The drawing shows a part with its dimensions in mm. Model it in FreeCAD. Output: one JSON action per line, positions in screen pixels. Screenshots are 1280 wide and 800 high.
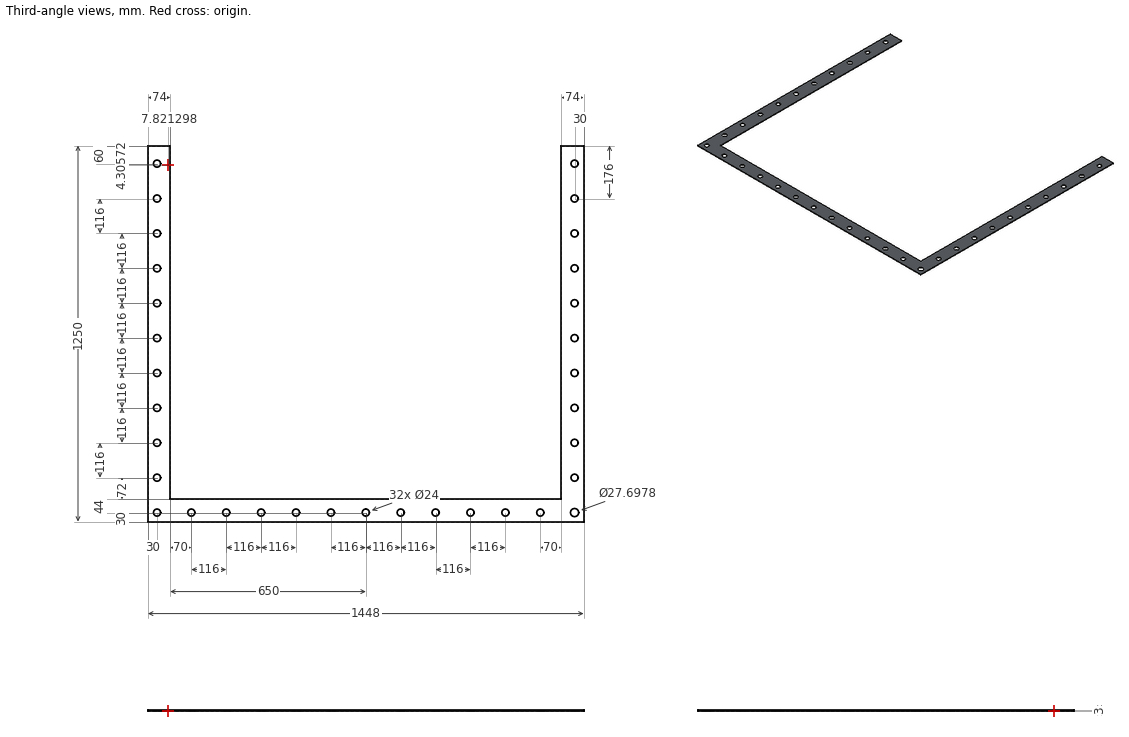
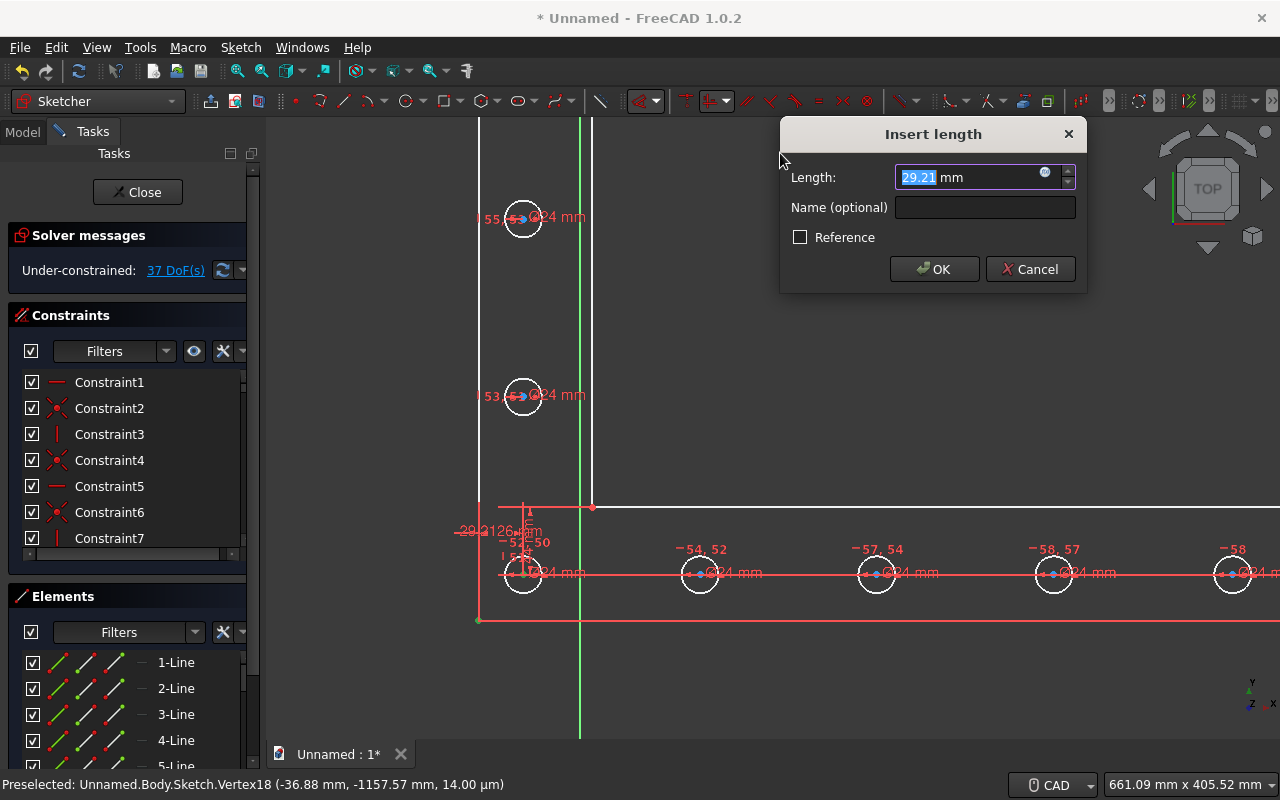
{"action": "type", "text": "30"}
{"action": "key", "text": "Return"}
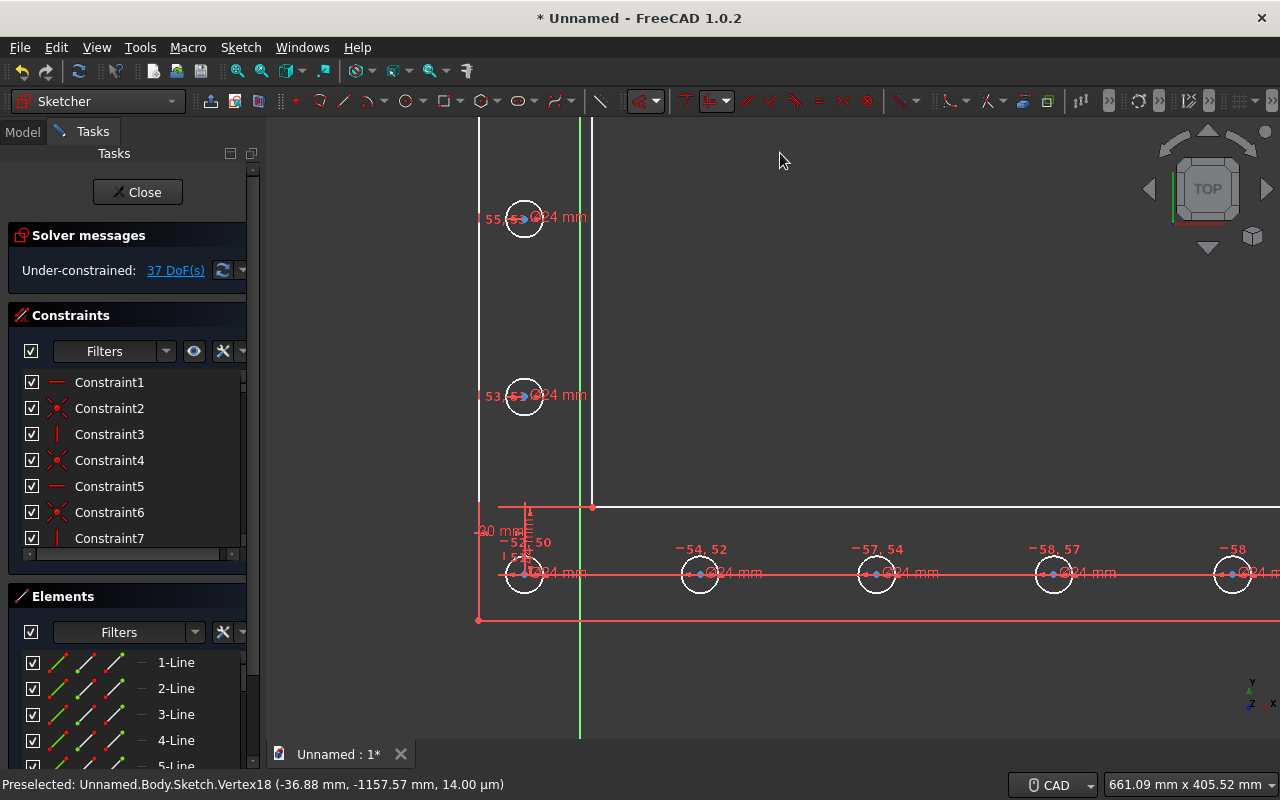
{"action": "left_click", "coordinate": [592, 507]}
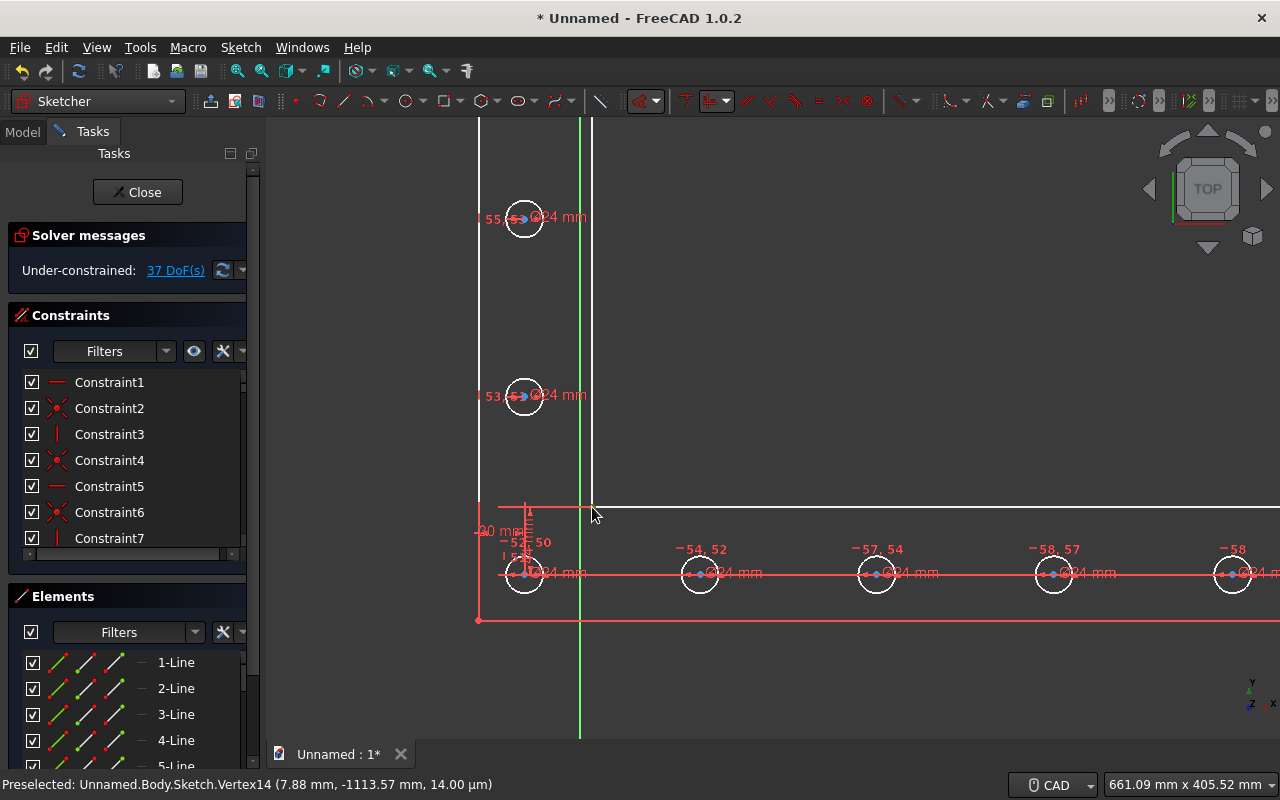
{"action": "left_click", "coordinate": [525, 397]}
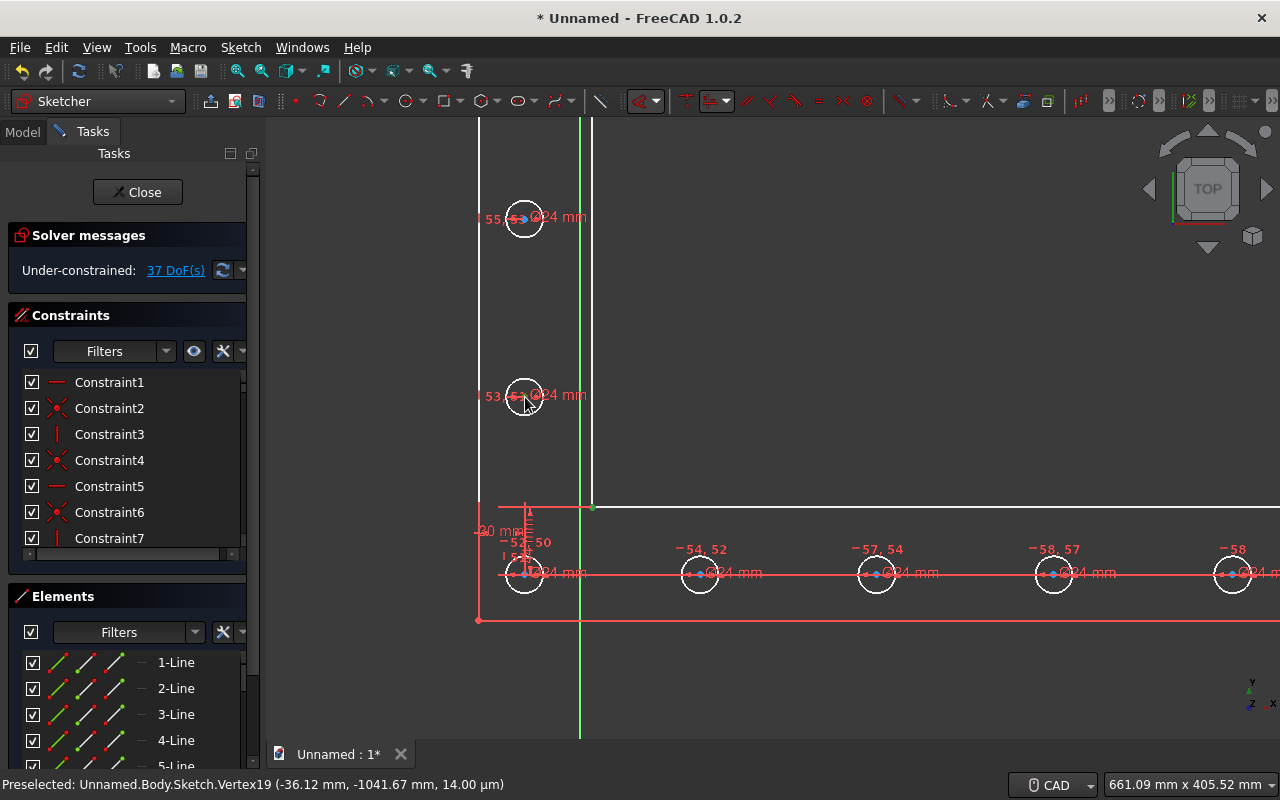
{"action": "left_click", "coordinate": [658, 102]}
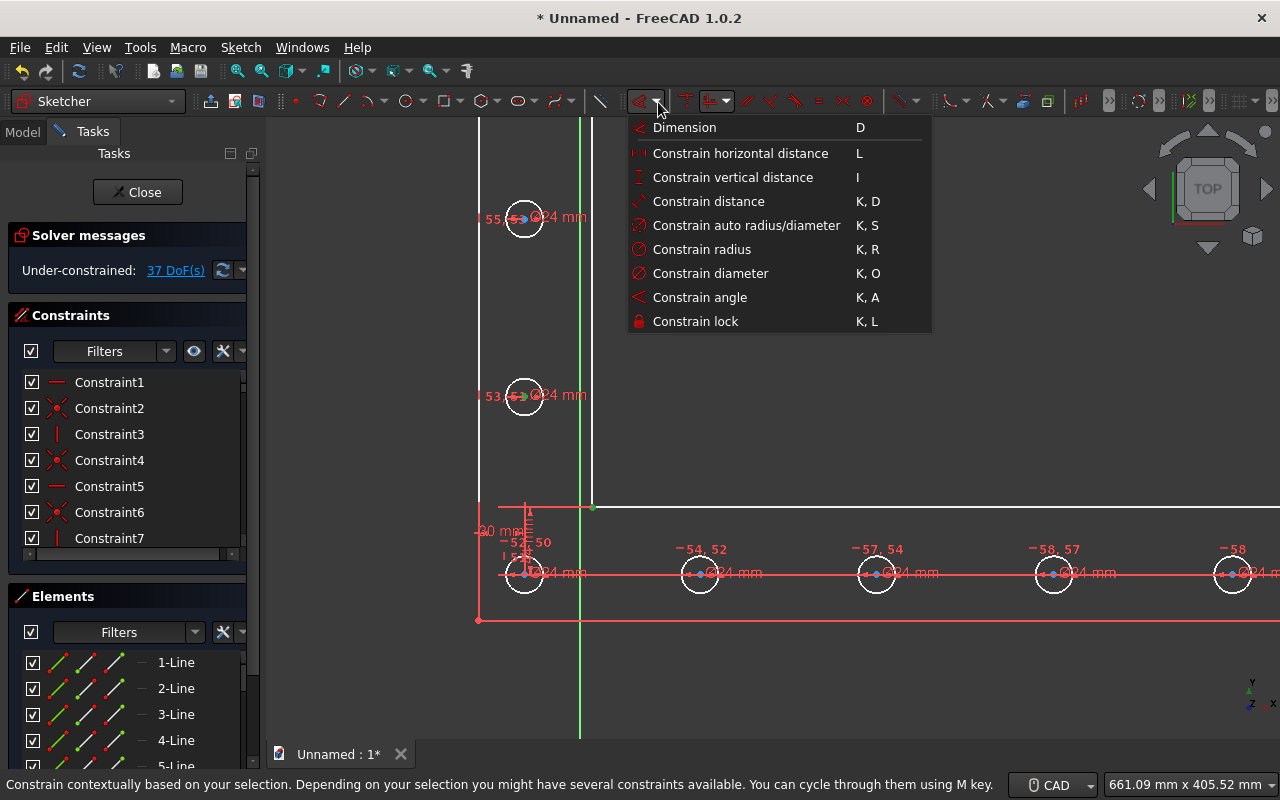
{"action": "left_click", "coordinate": [780, 177]}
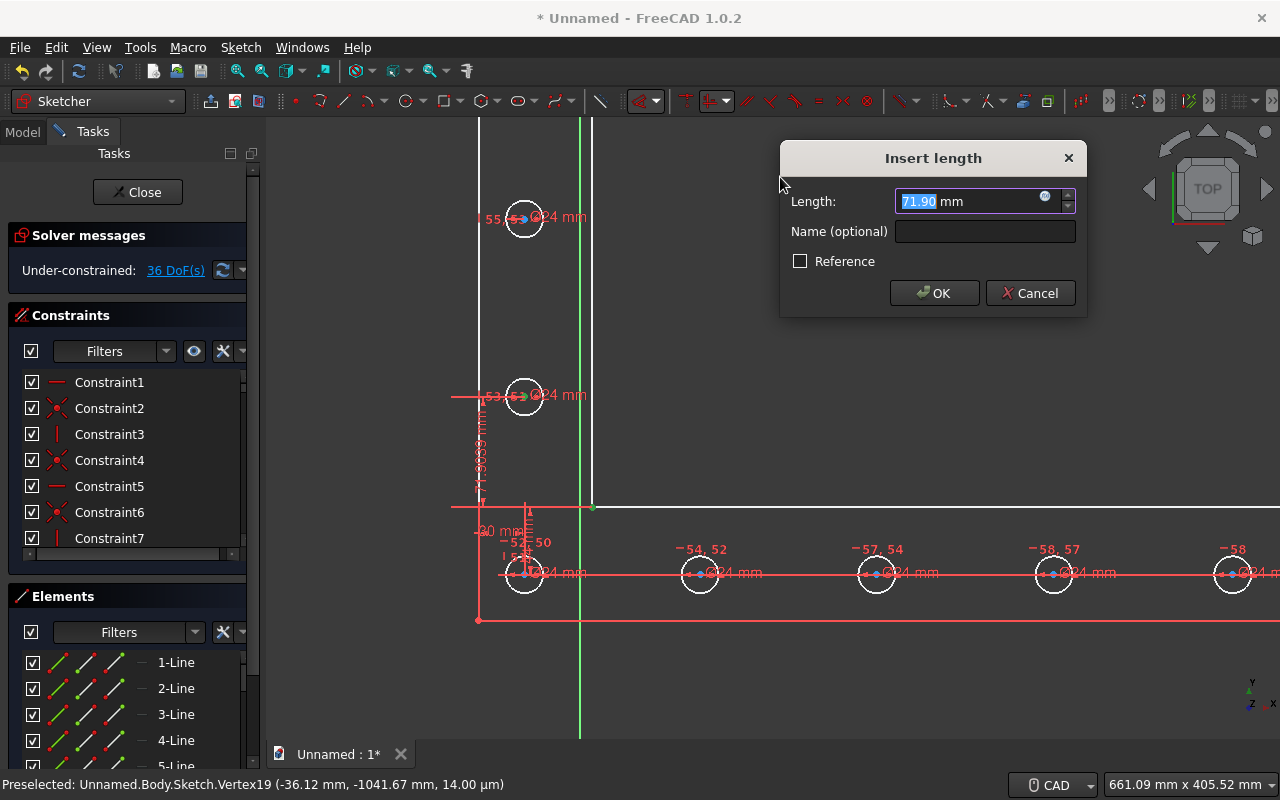
{"action": "type", "text": "72"}
{"action": "key", "text": "Return"}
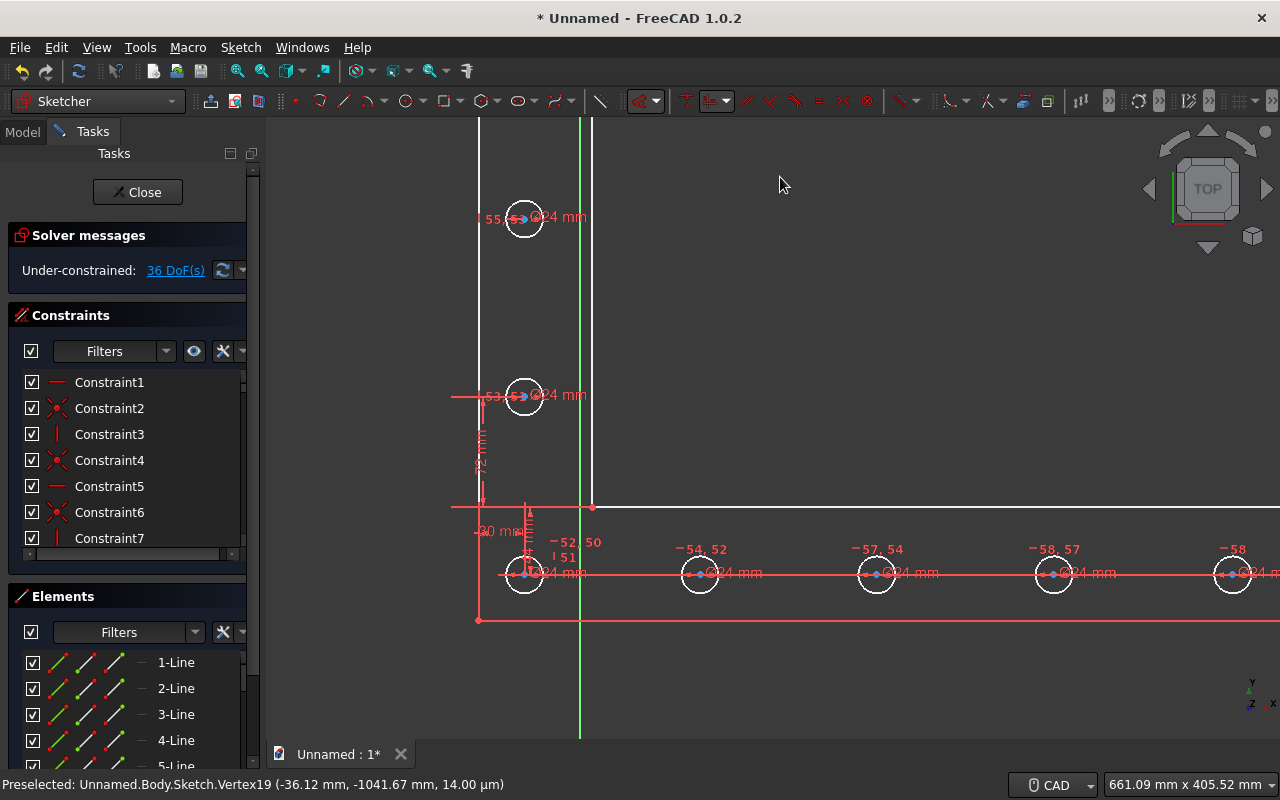
{"action": "left_click", "coordinate": [592, 507]}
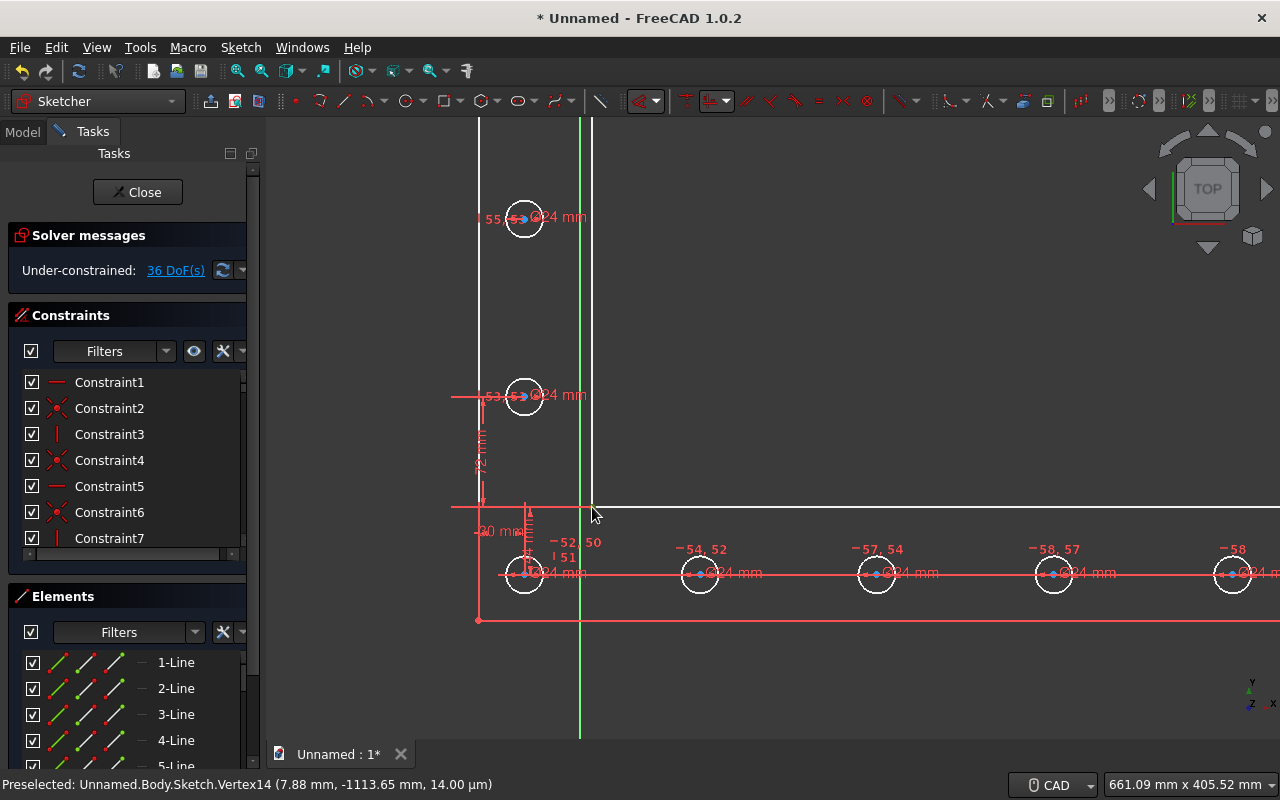
{"action": "left_click", "coordinate": [700, 575]}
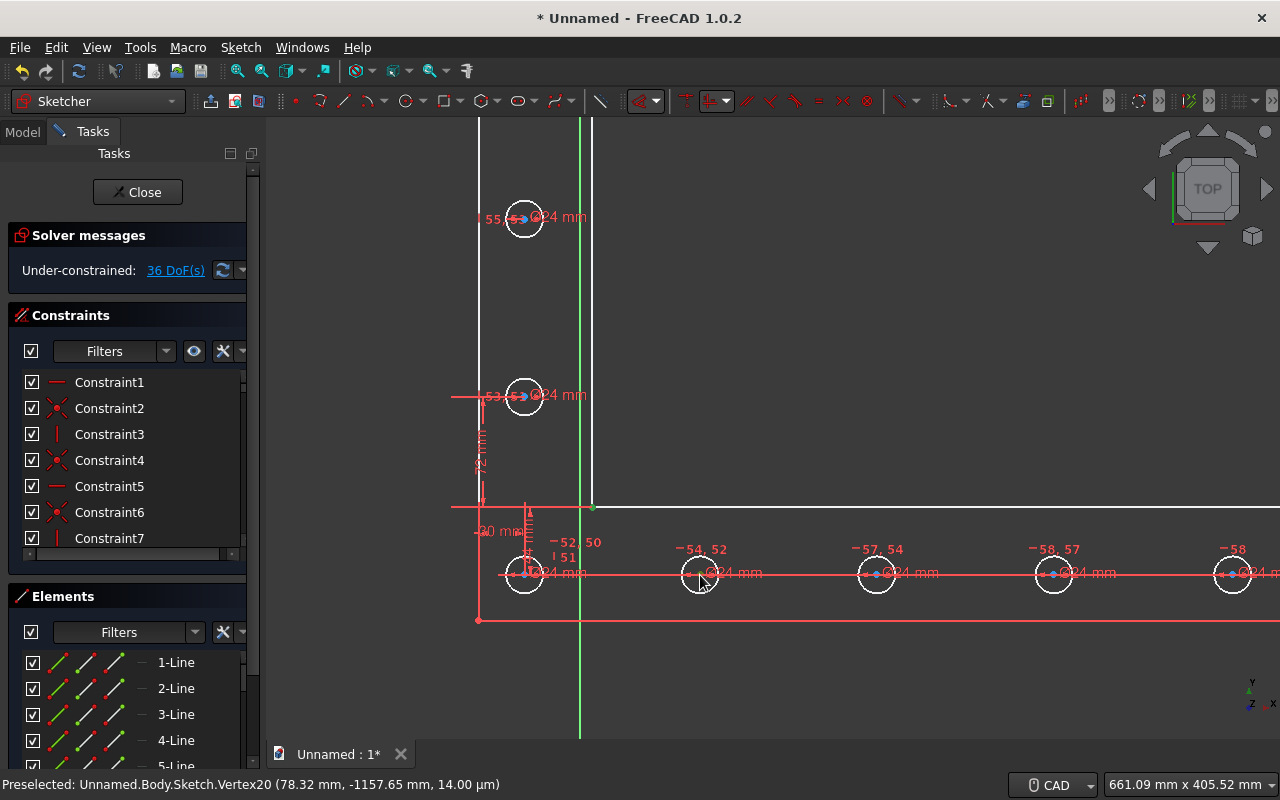
{"action": "left_click", "coordinate": [658, 102]}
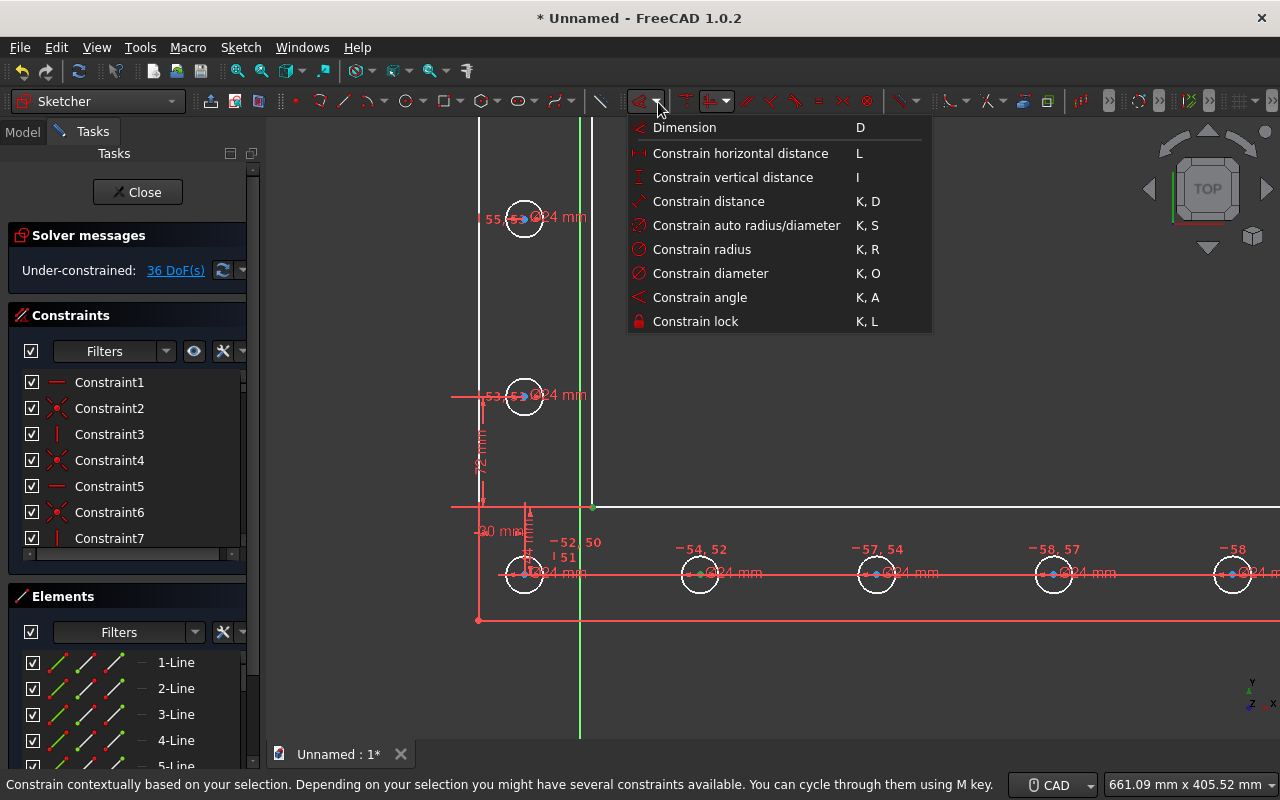
{"action": "left_click", "coordinate": [780, 153]}